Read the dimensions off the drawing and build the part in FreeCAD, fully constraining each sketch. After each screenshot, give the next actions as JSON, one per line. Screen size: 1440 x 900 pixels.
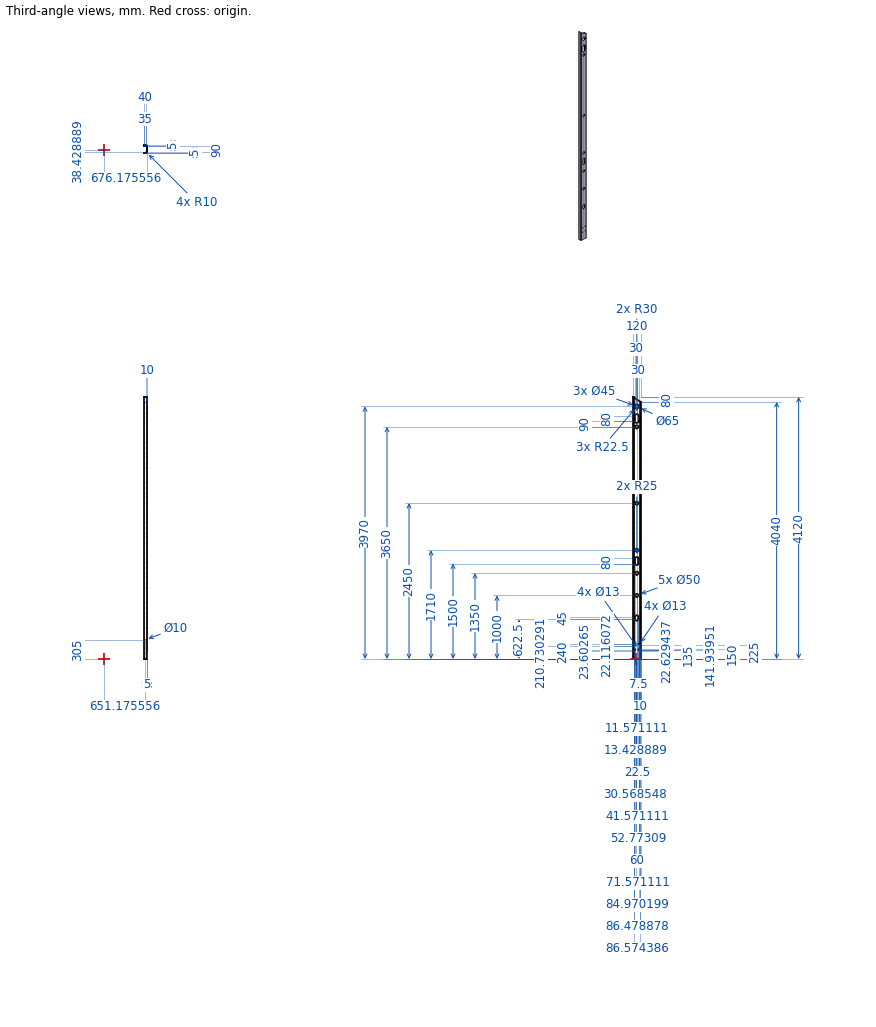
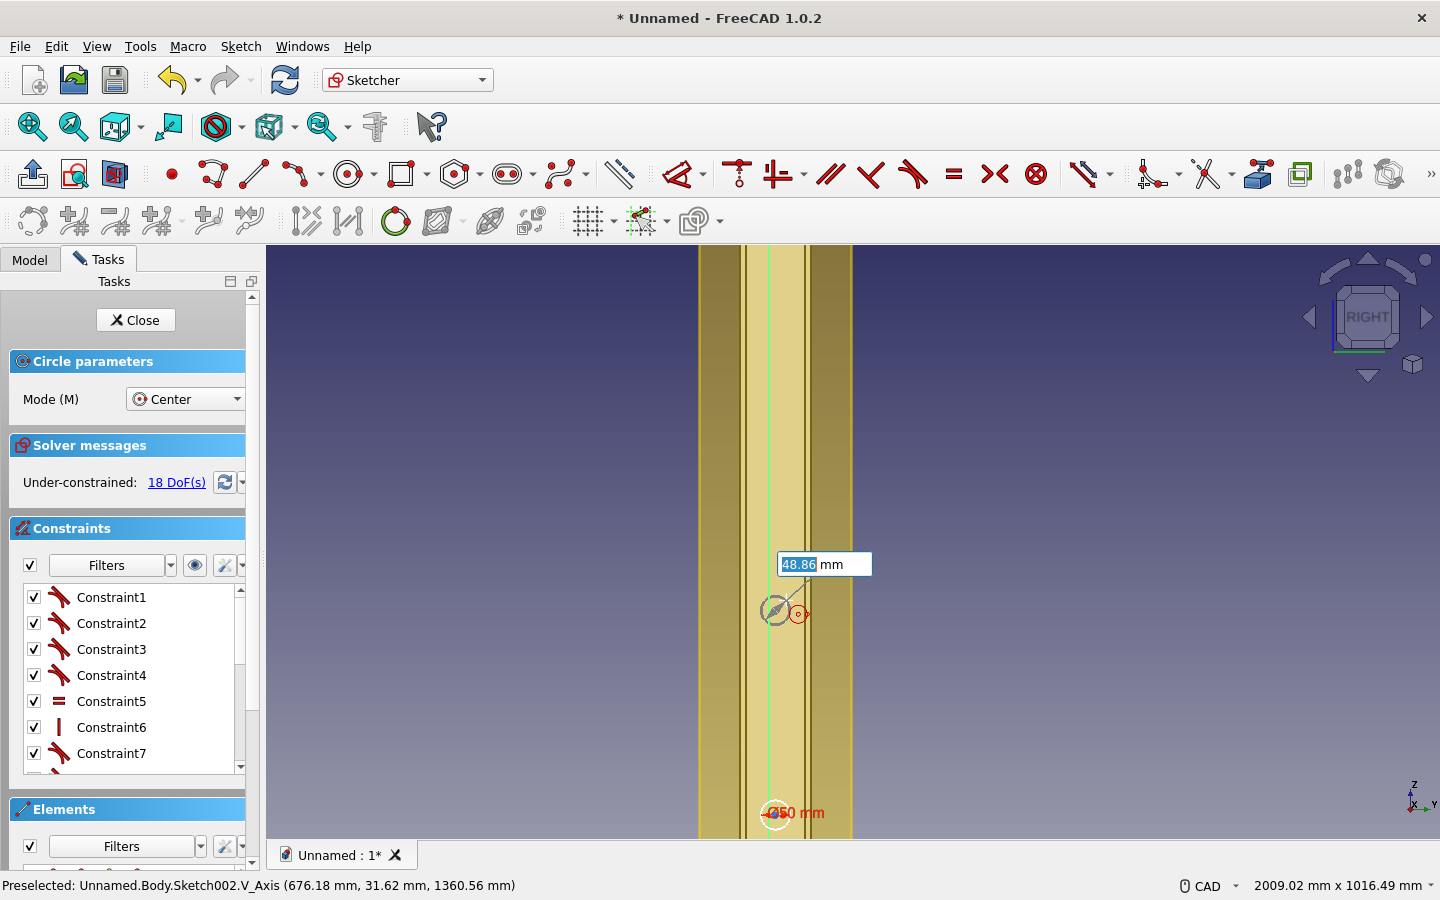
{"action": "type", "text": "50"}
{"action": "key", "text": "Return"}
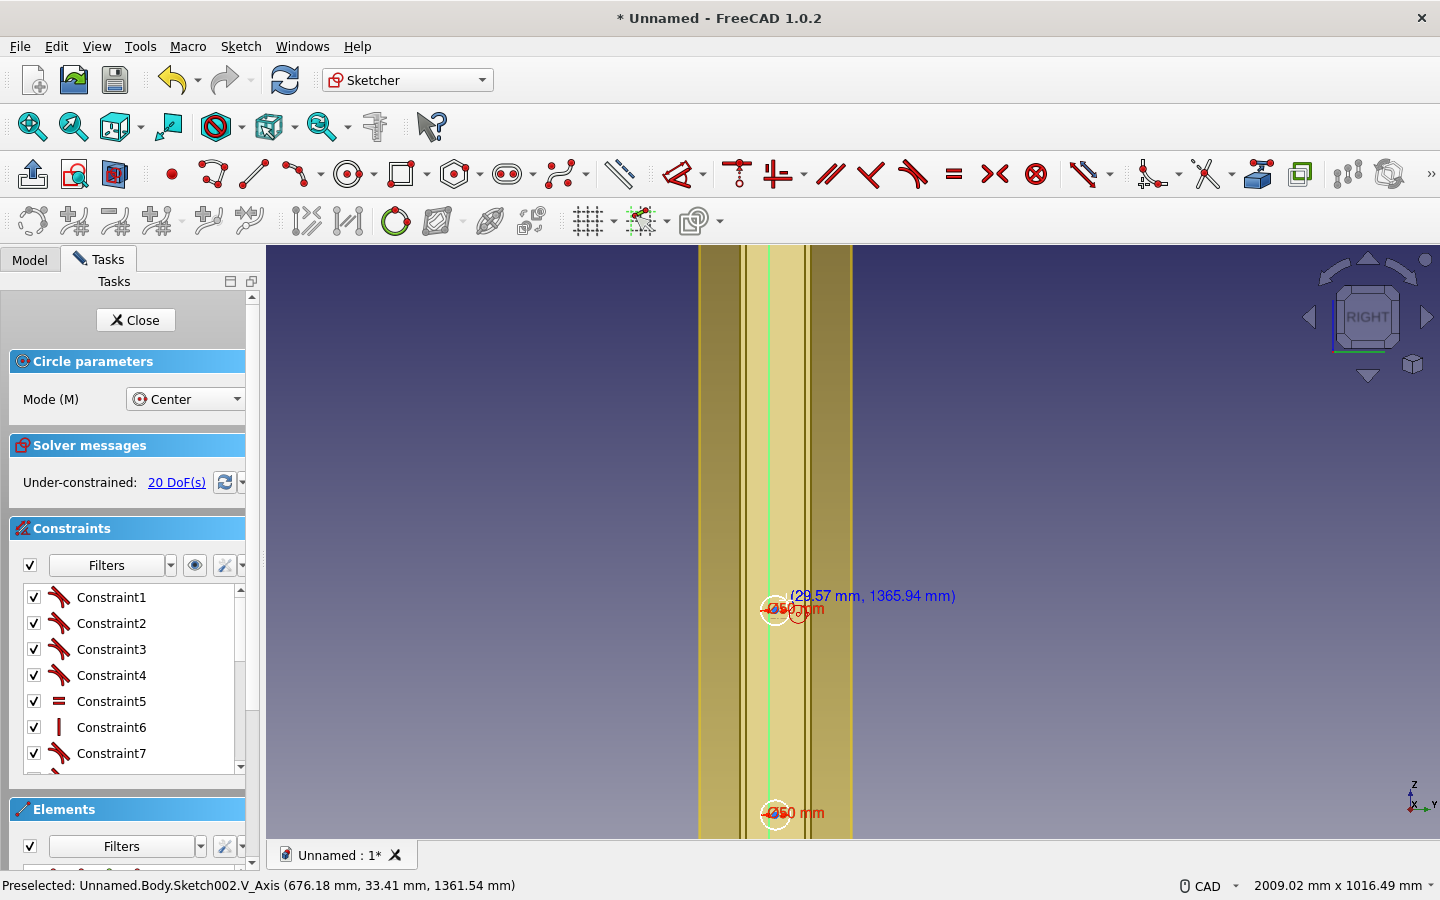
{"action": "scroll", "coordinate": [786, 603], "scroll_direction": "down", "scroll_amount": 9}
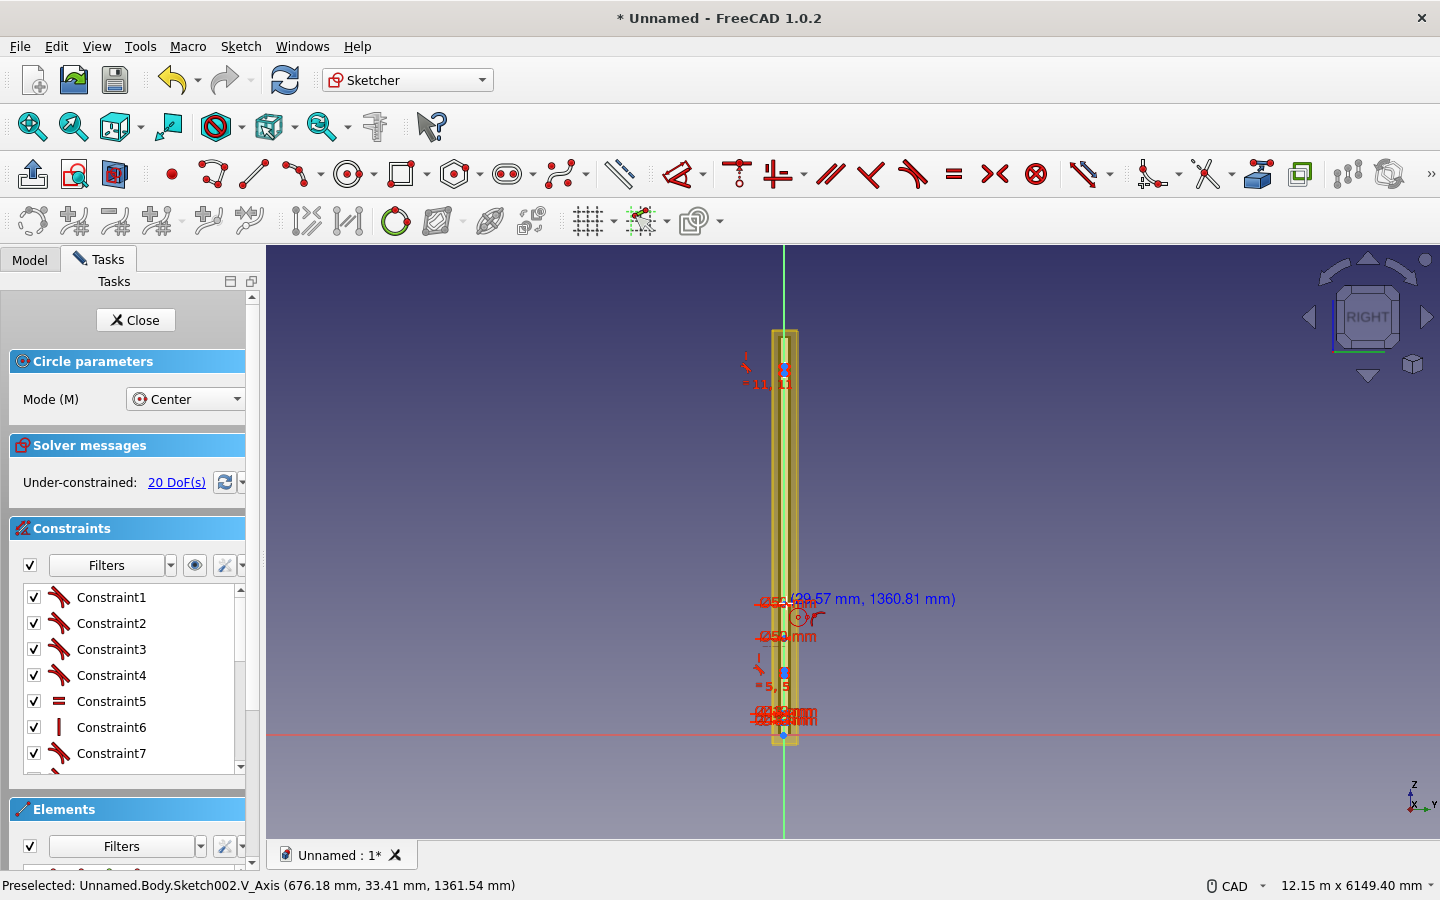
{"action": "scroll", "coordinate": [785, 352], "scroll_direction": "up", "scroll_amount": 14}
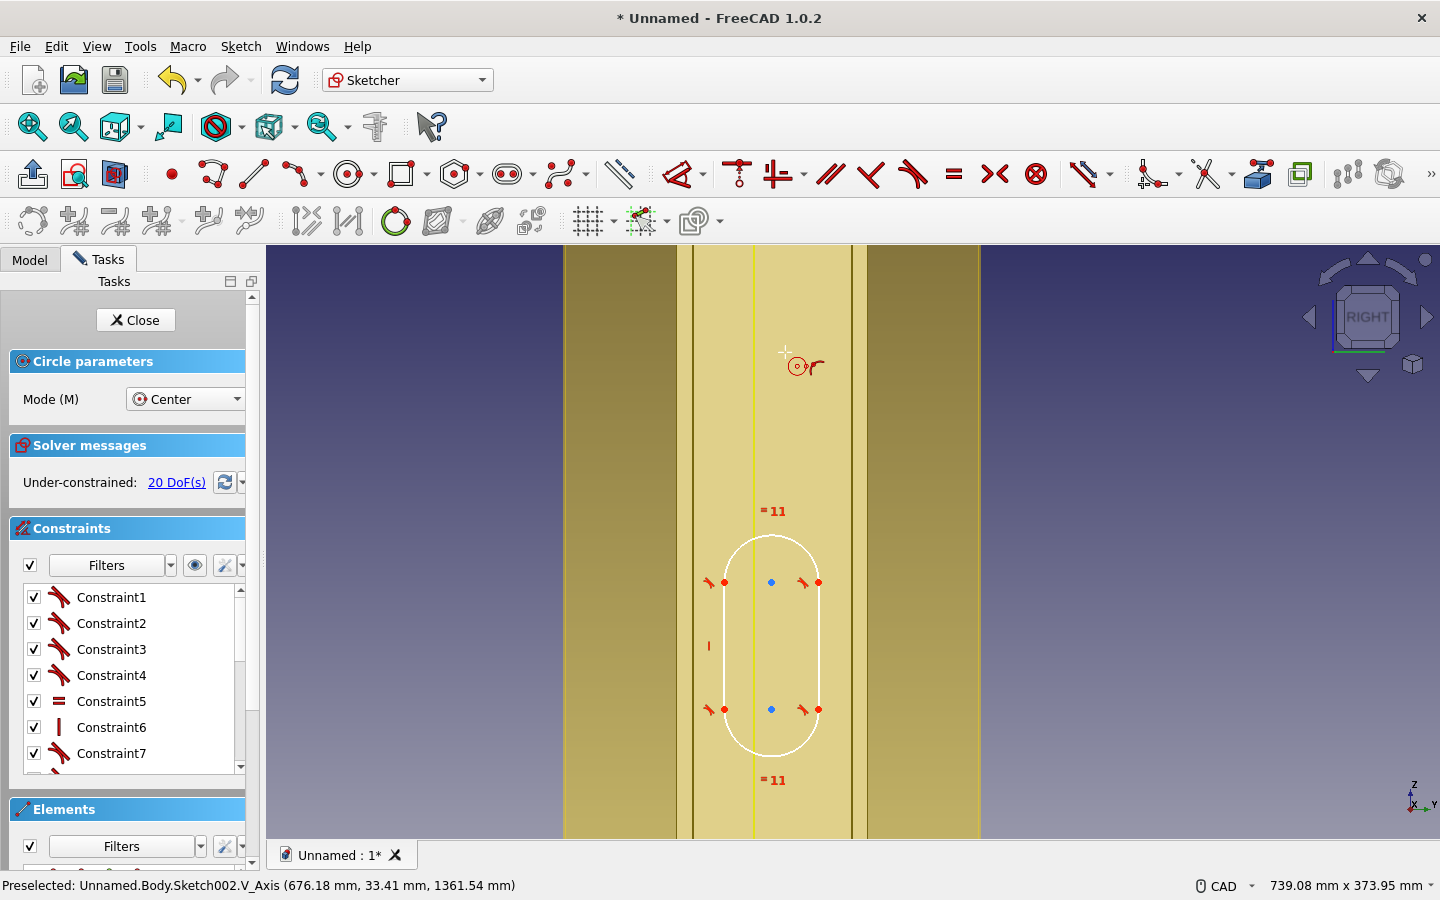
{"action": "left_click", "coordinate": [772, 343]}
{"action": "mouse_move", "coordinate": [797, 318]}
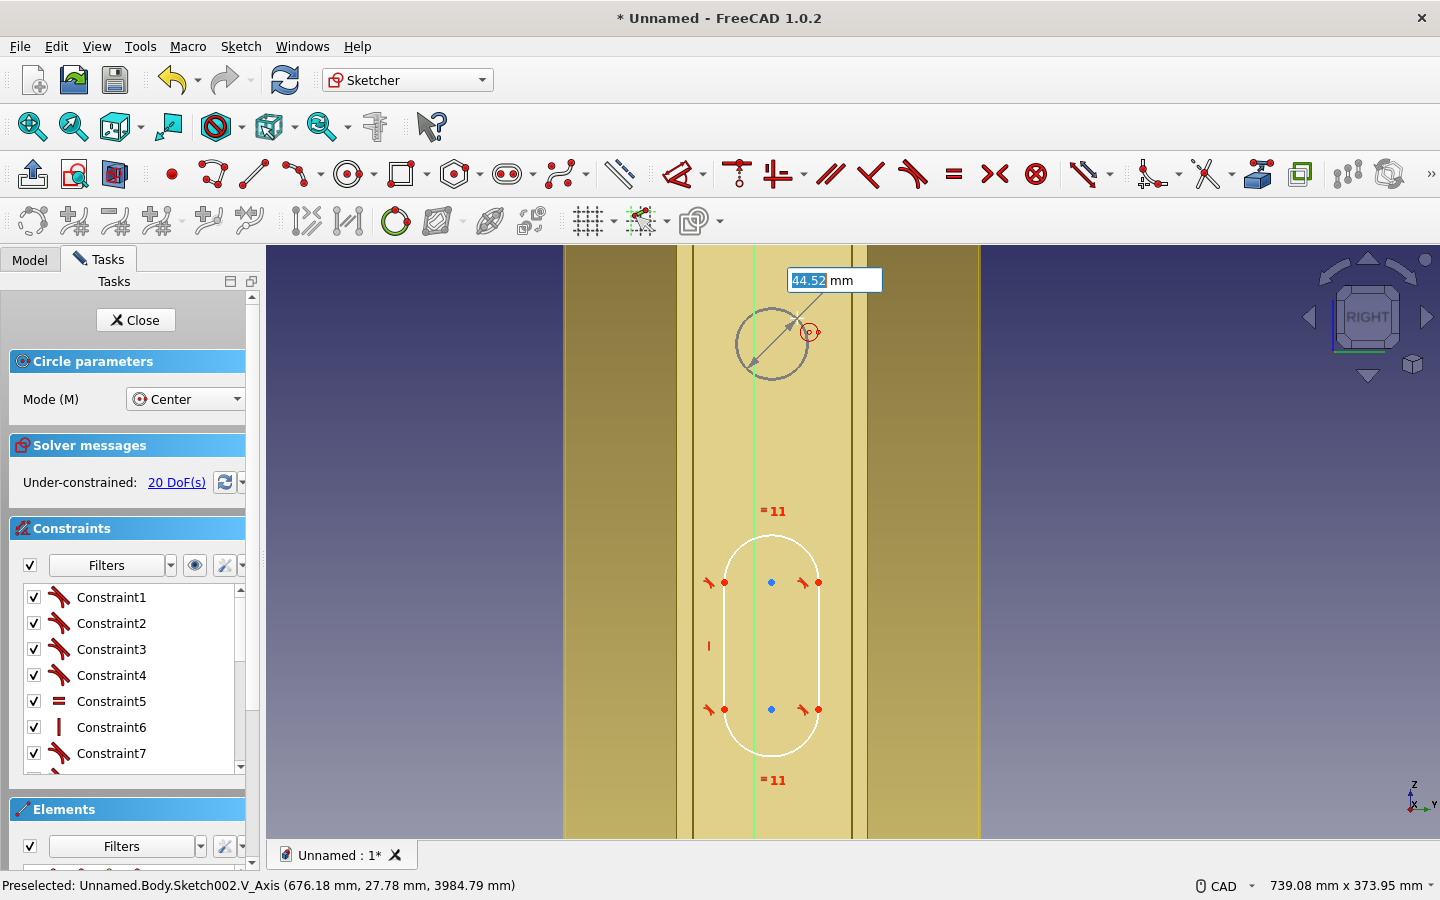
{"action": "type", "text": "45"}
{"action": "key", "text": "Return"}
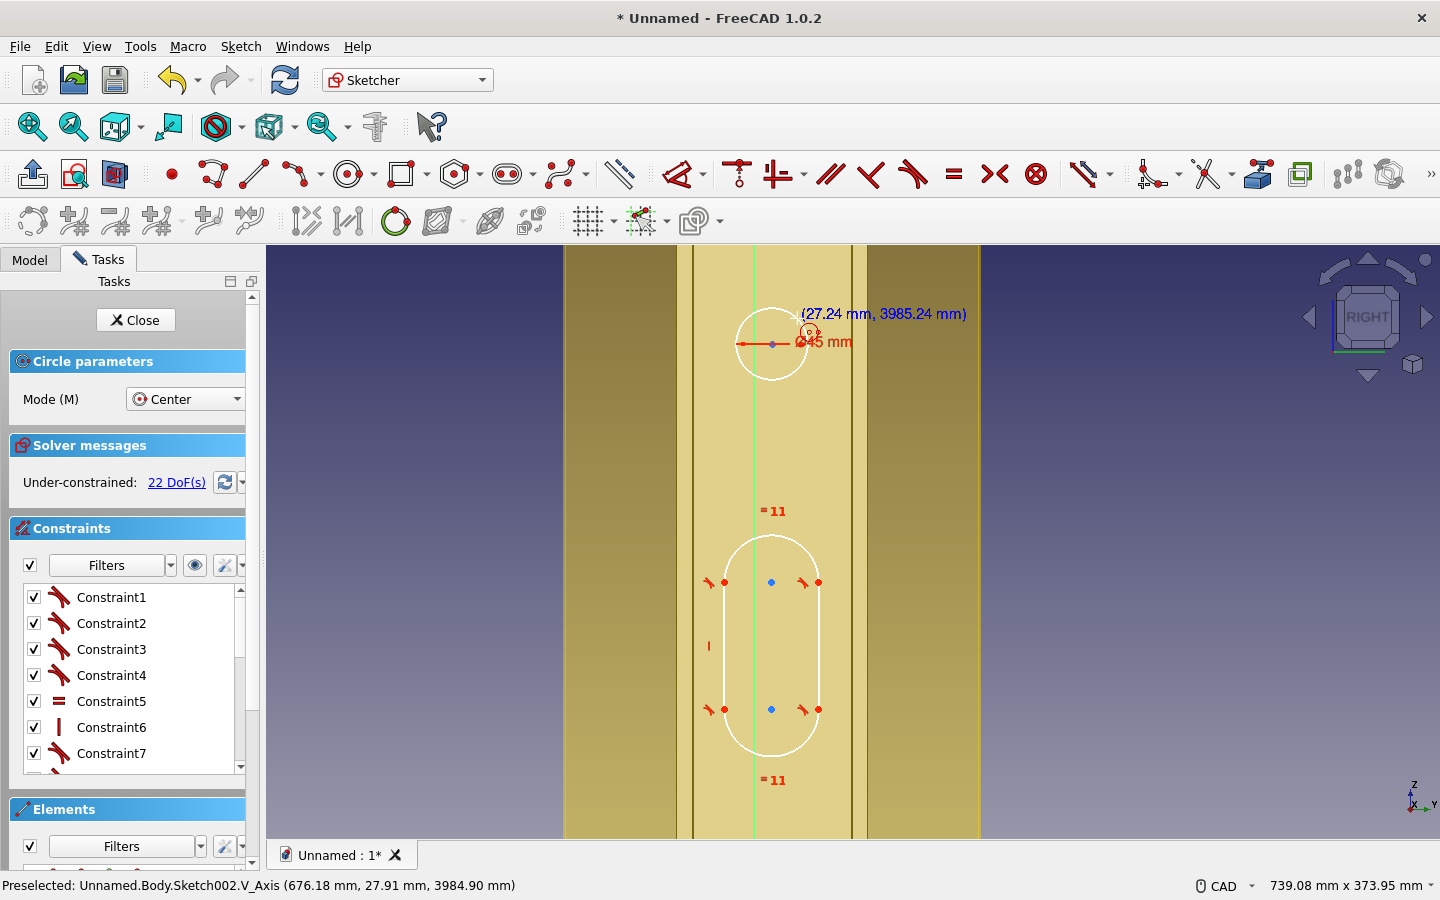
{"action": "scroll", "coordinate": [785, 352], "scroll_direction": "down", "scroll_amount": 14}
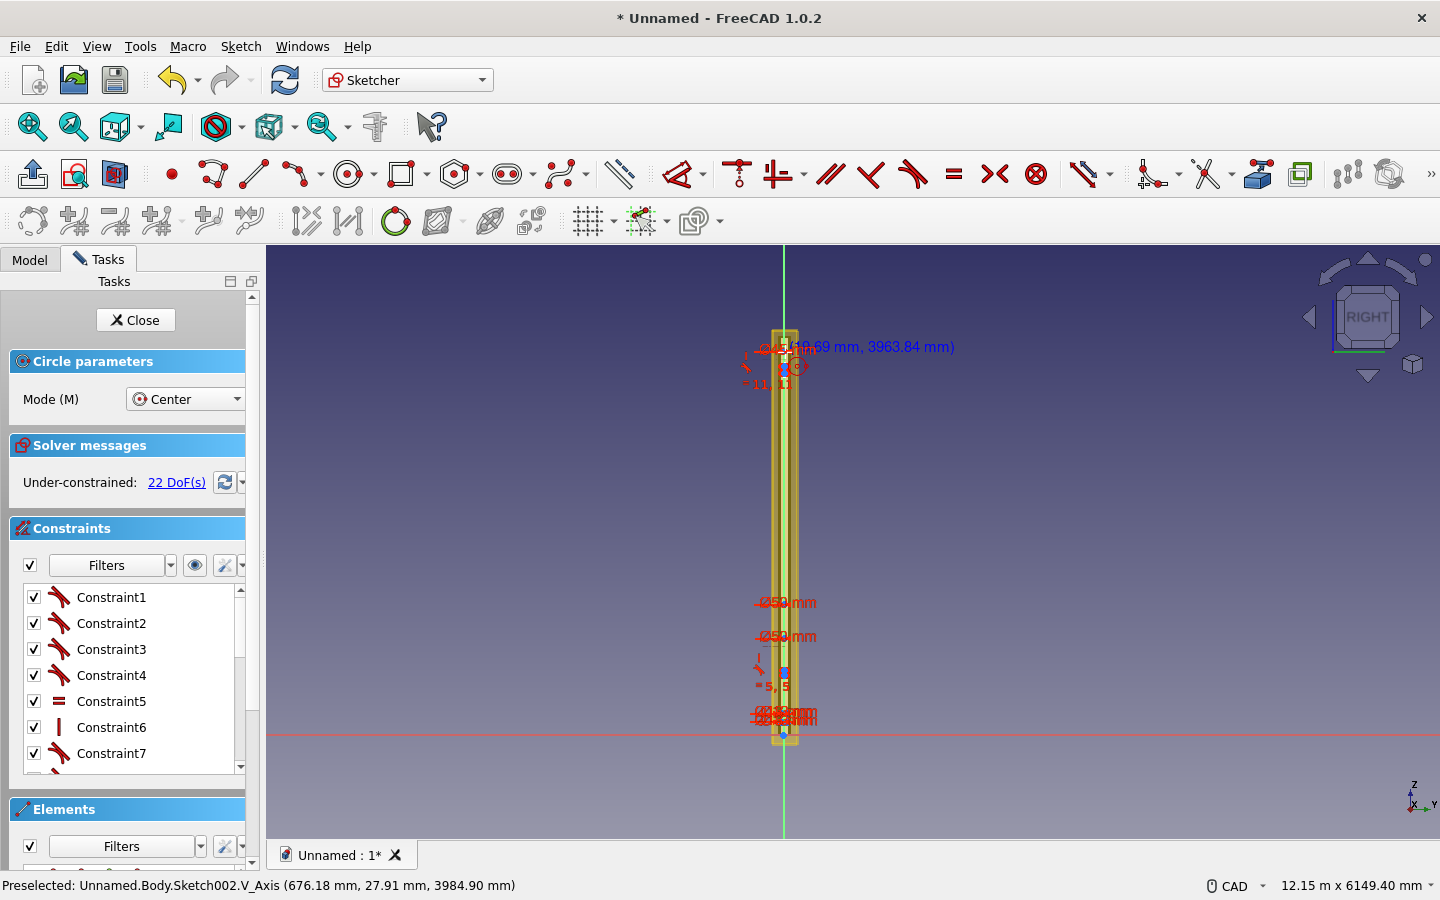
{"action": "scroll", "coordinate": [785, 383], "scroll_direction": "up", "scroll_amount": 14}